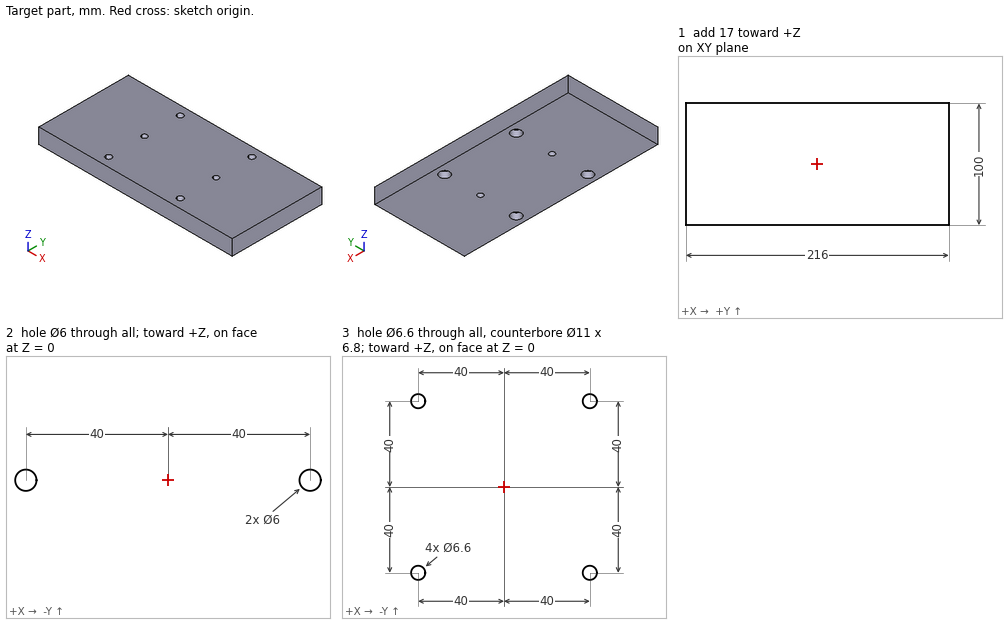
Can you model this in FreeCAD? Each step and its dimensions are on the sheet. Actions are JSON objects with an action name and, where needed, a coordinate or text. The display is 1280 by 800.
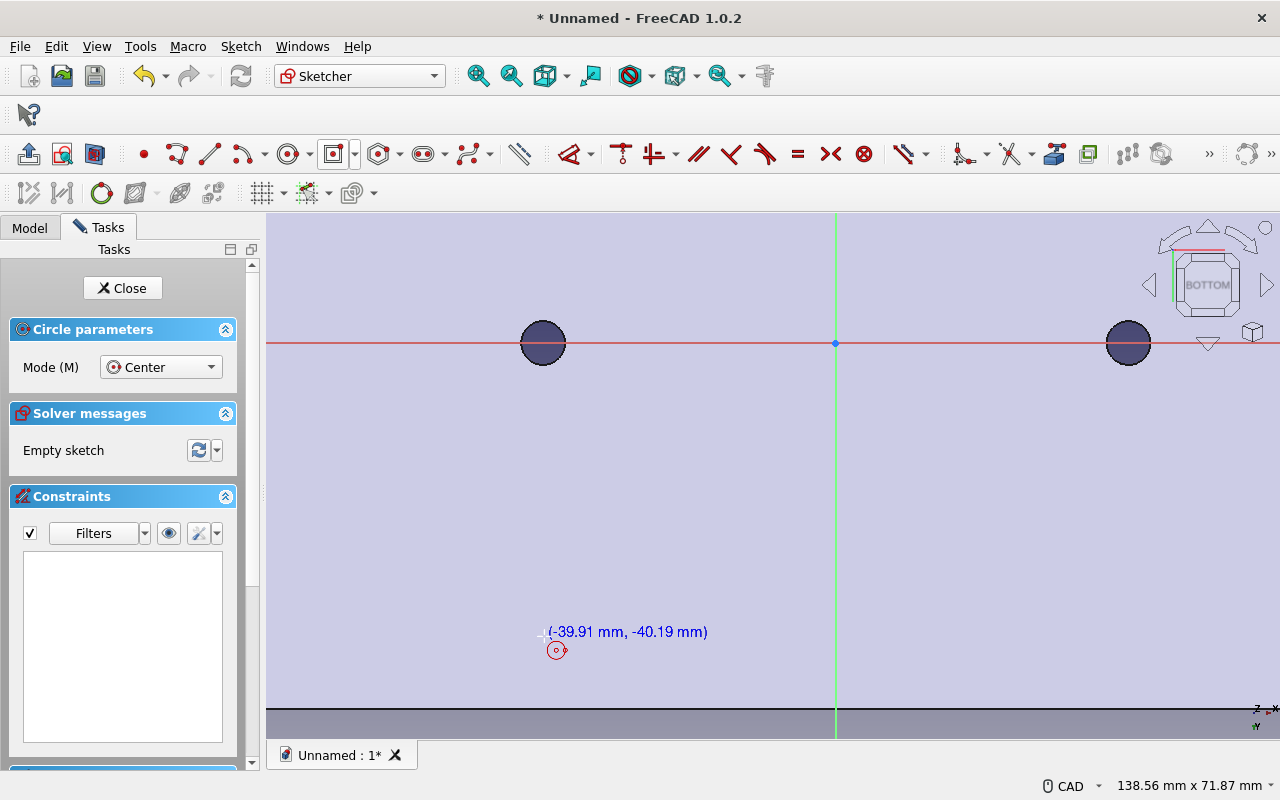
{"action": "left_click", "coordinate": [543, 636]}
{"action": "mouse_move", "coordinate": [560, 619]}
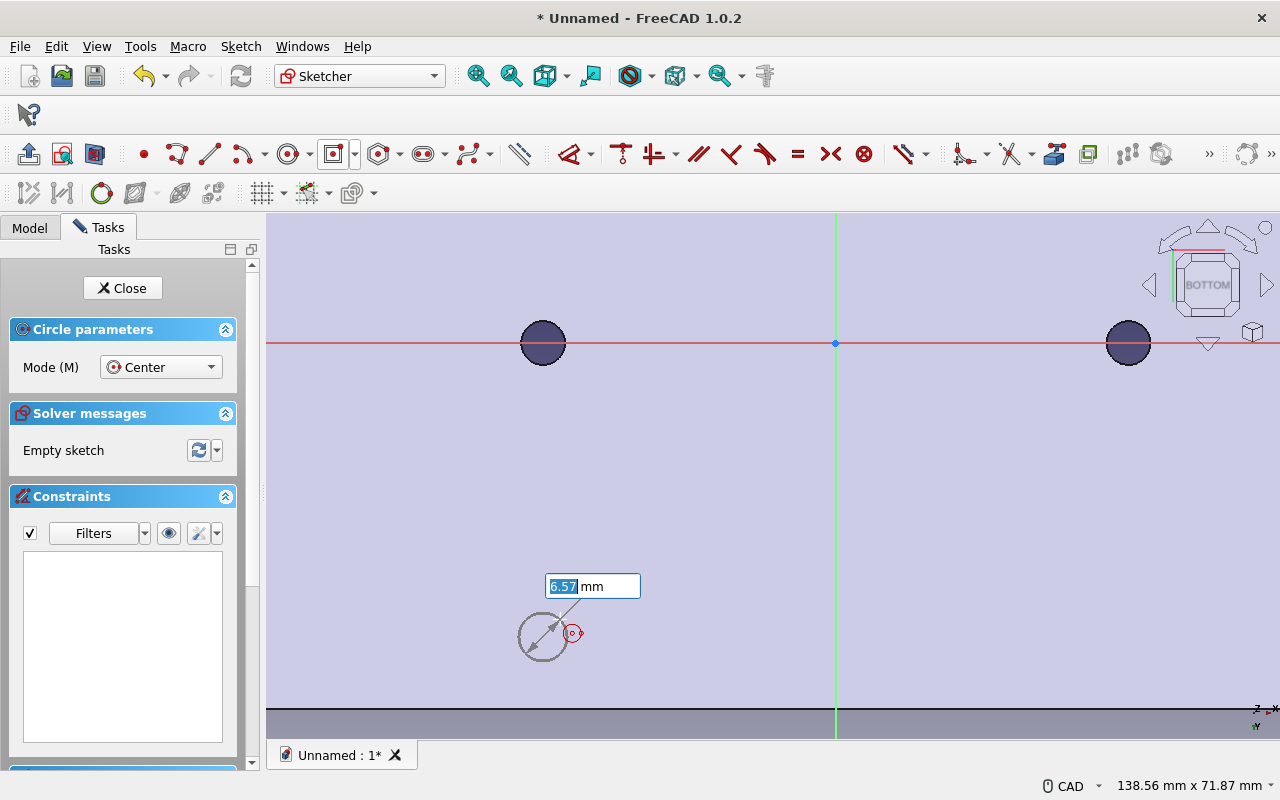
{"action": "type", "text": "6.6"}
{"action": "key", "text": "Return"}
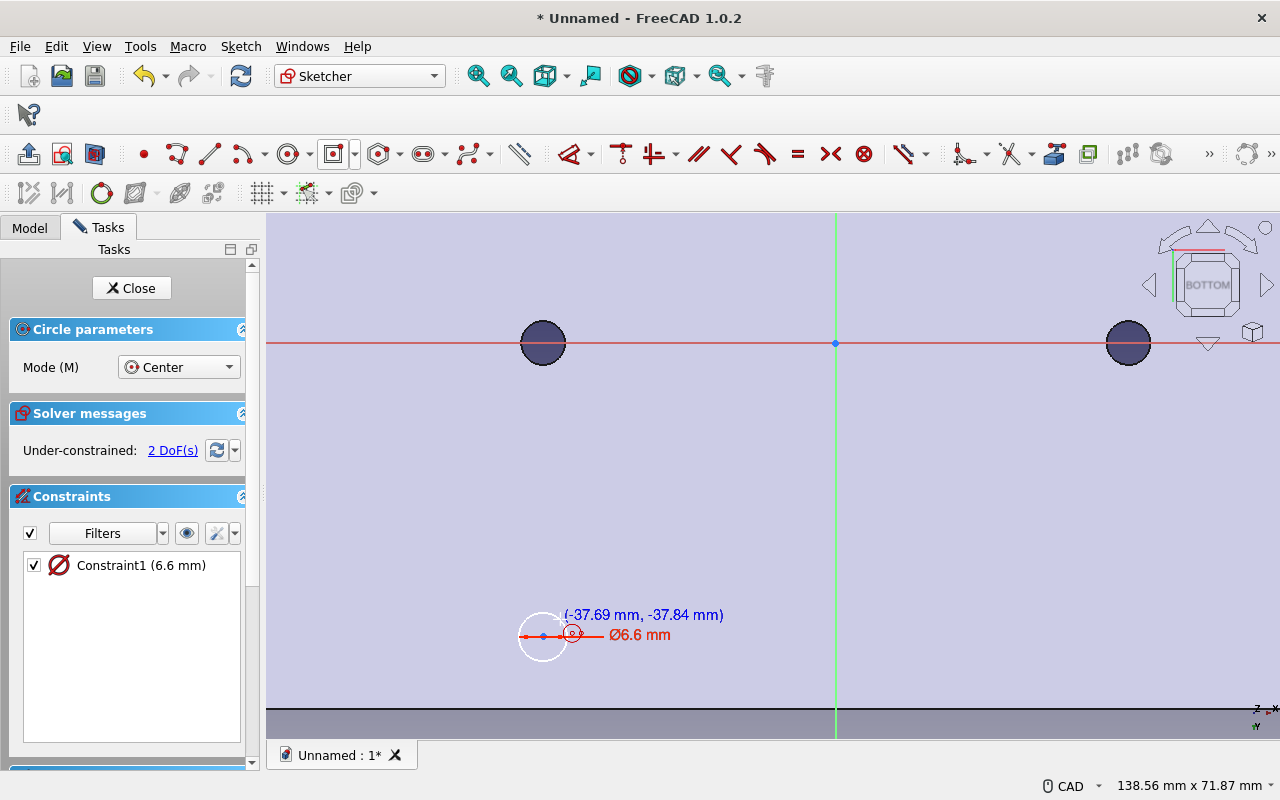
{"action": "scroll", "coordinate": [545, 638], "scroll_direction": "down", "scroll_amount": 3}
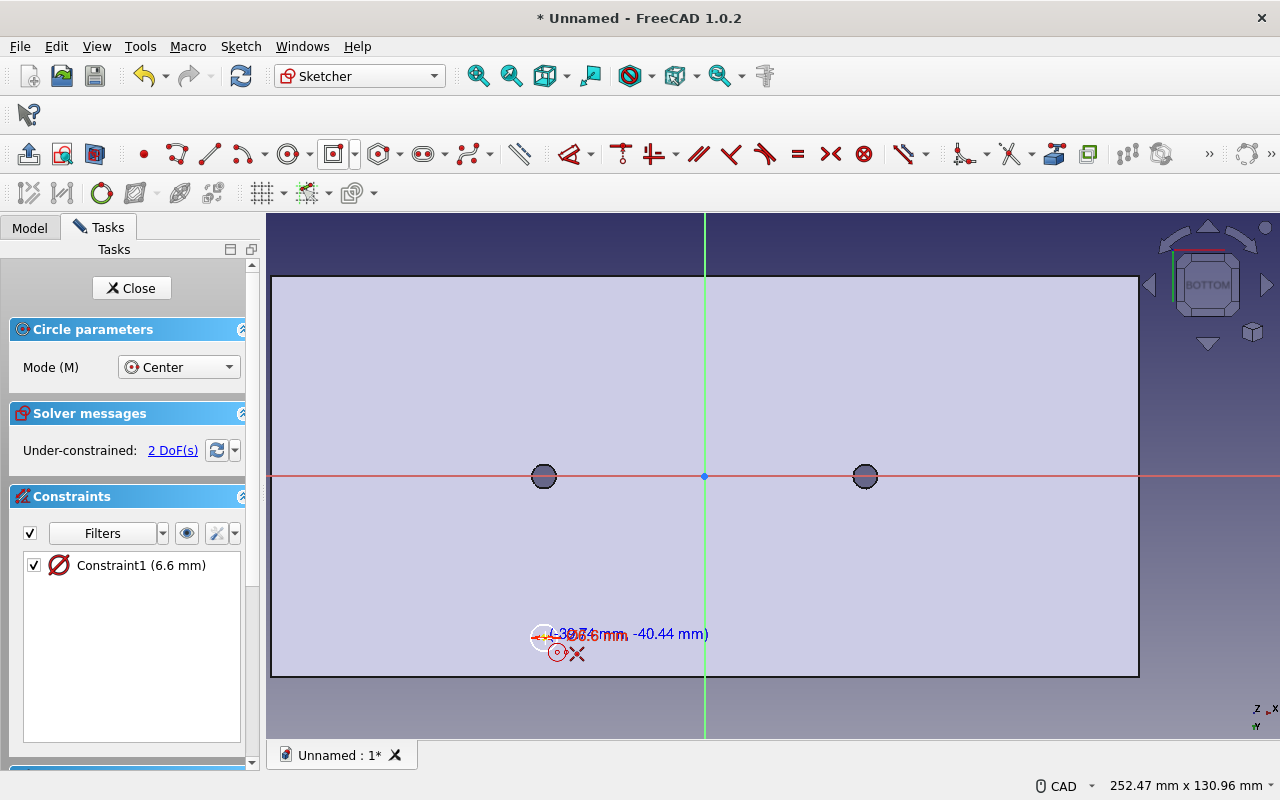
{"action": "scroll", "coordinate": [544, 316], "scroll_direction": "up", "scroll_amount": 3}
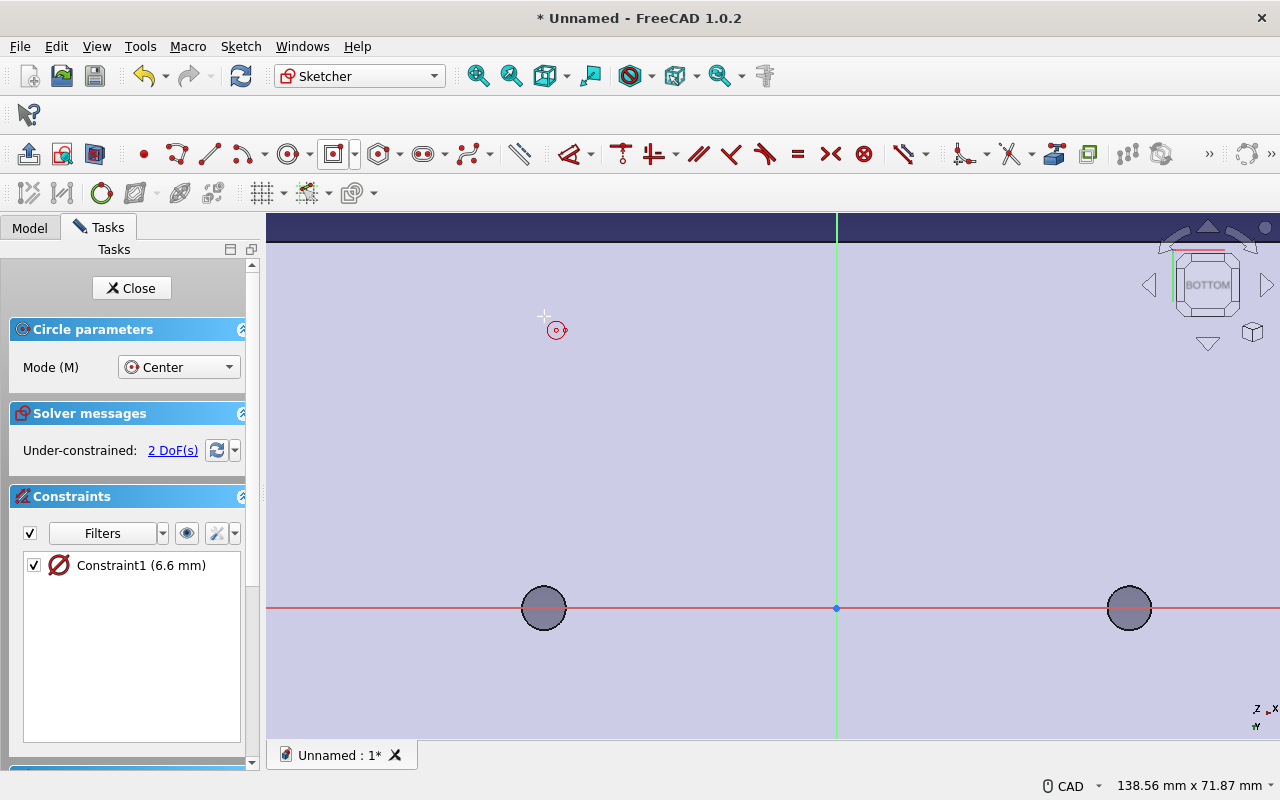
{"action": "left_click", "coordinate": [544, 316]}
{"action": "mouse_move", "coordinate": [561, 298]}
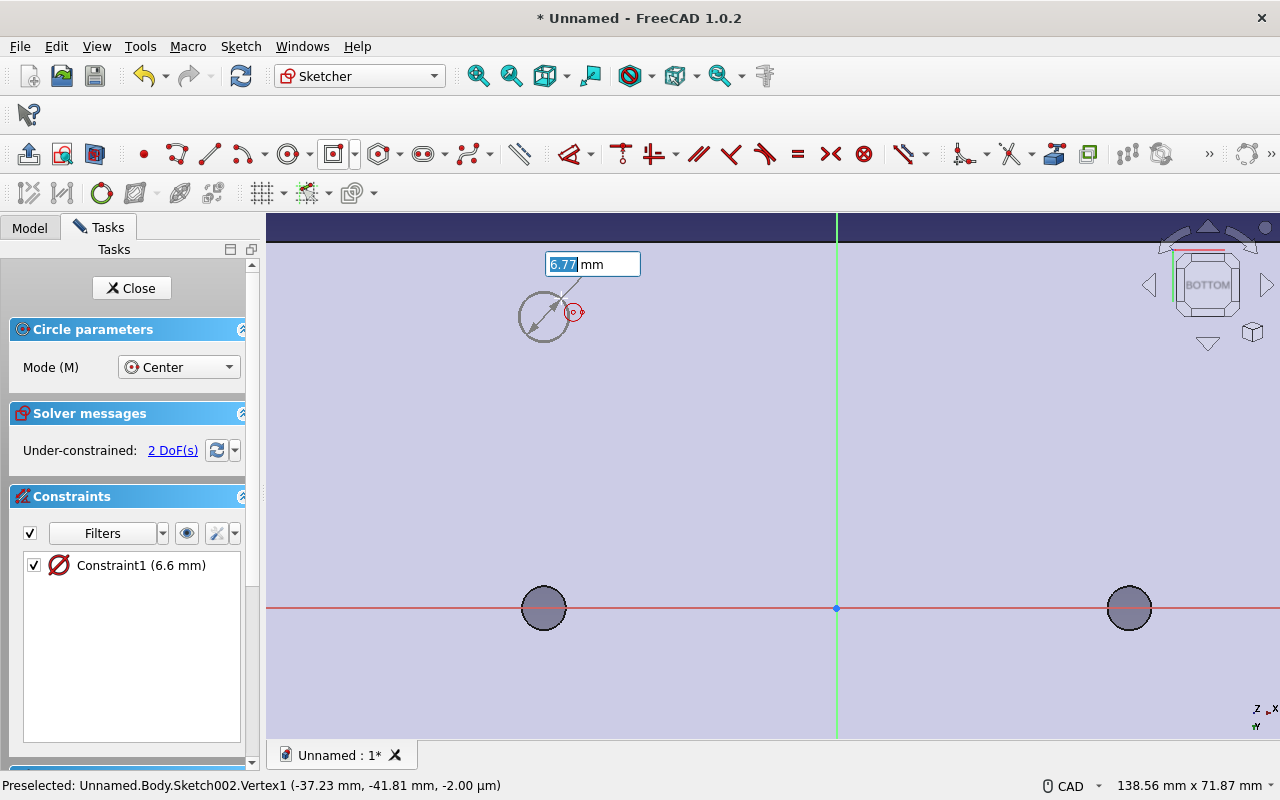
{"action": "type", "text": "6.6"}
{"action": "key", "text": "Return"}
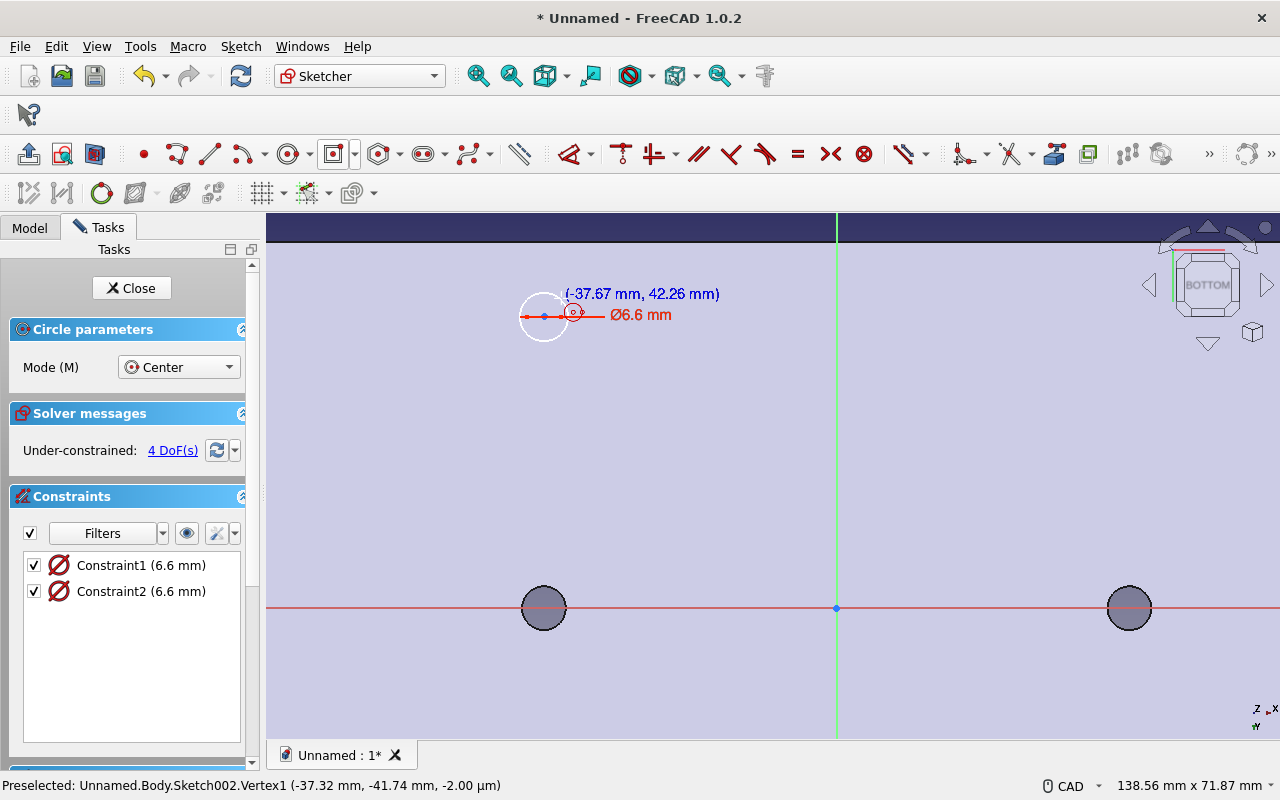
{"action": "scroll", "coordinate": [544, 315], "scroll_direction": "down", "scroll_amount": 3}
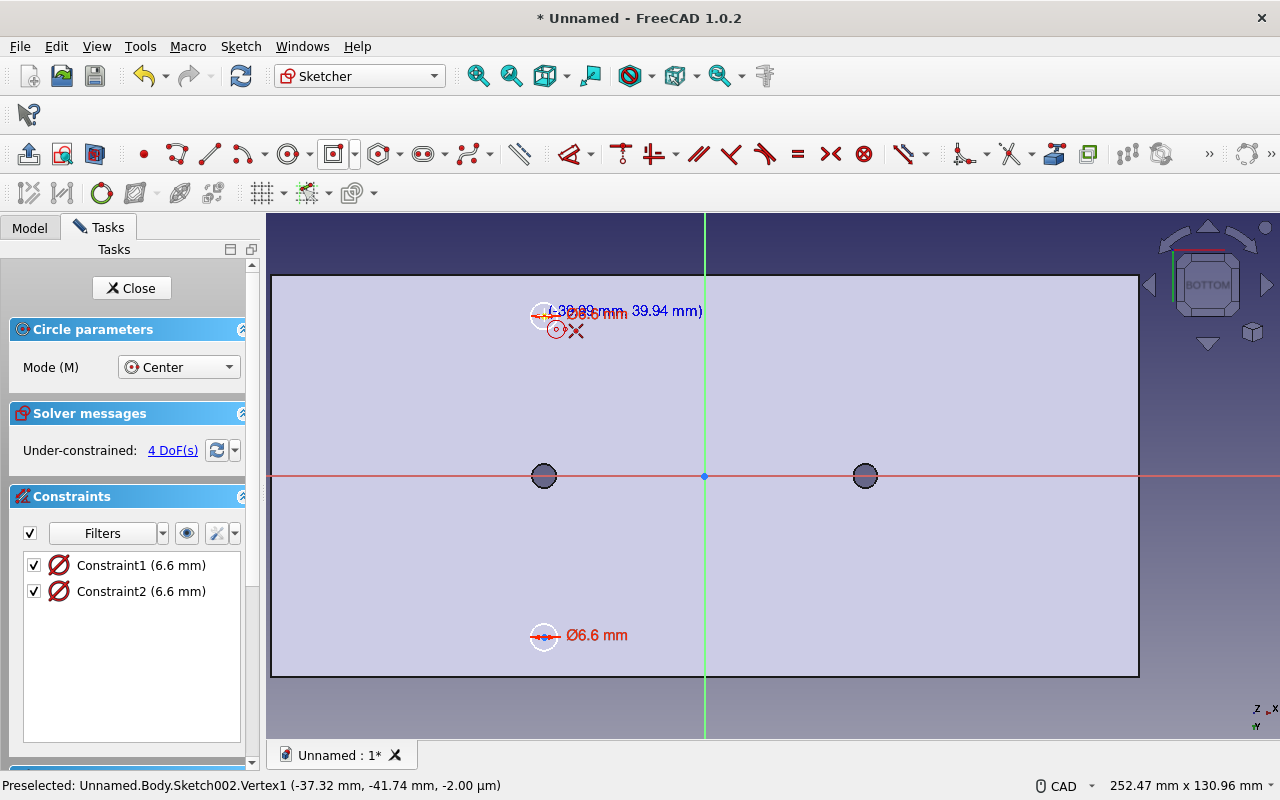
{"action": "scroll", "coordinate": [865, 315], "scroll_direction": "up", "scroll_amount": 3}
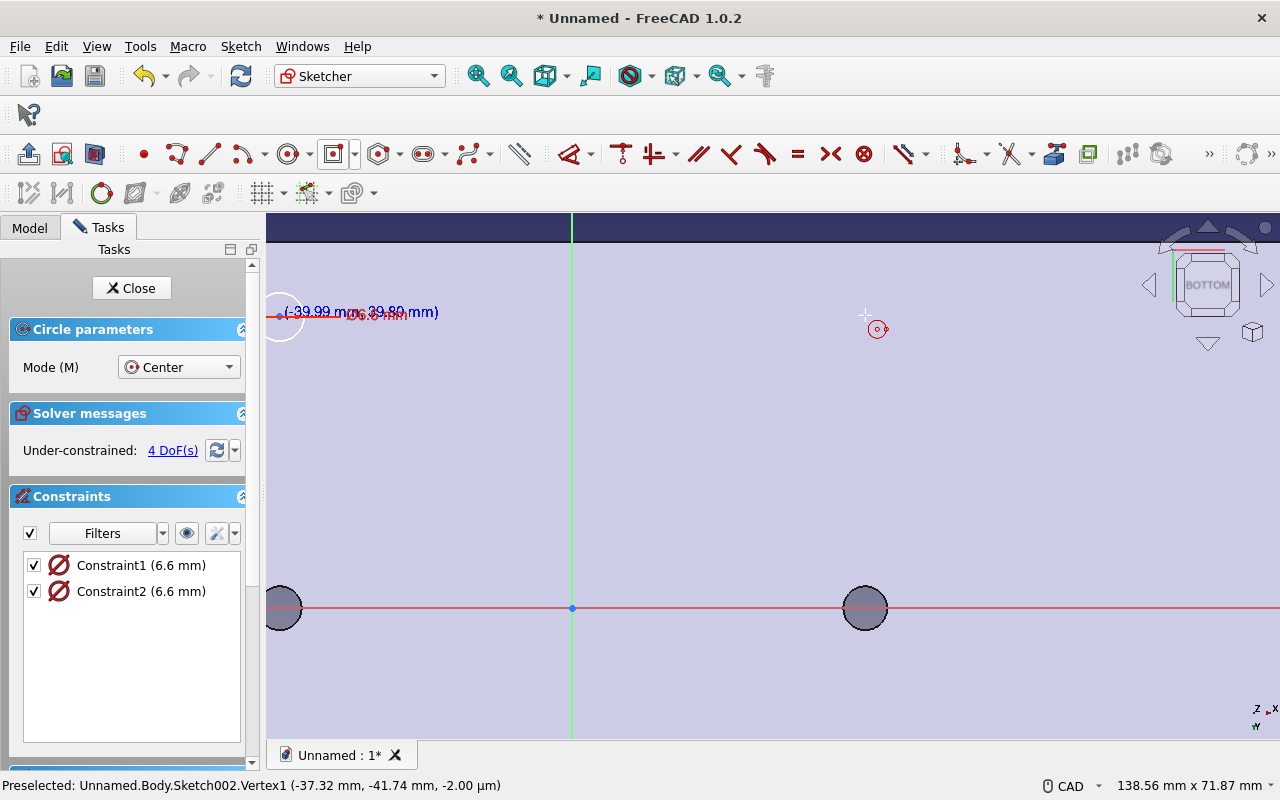
{"action": "left_click", "coordinate": [865, 316]}
{"action": "mouse_move", "coordinate": [882, 298]}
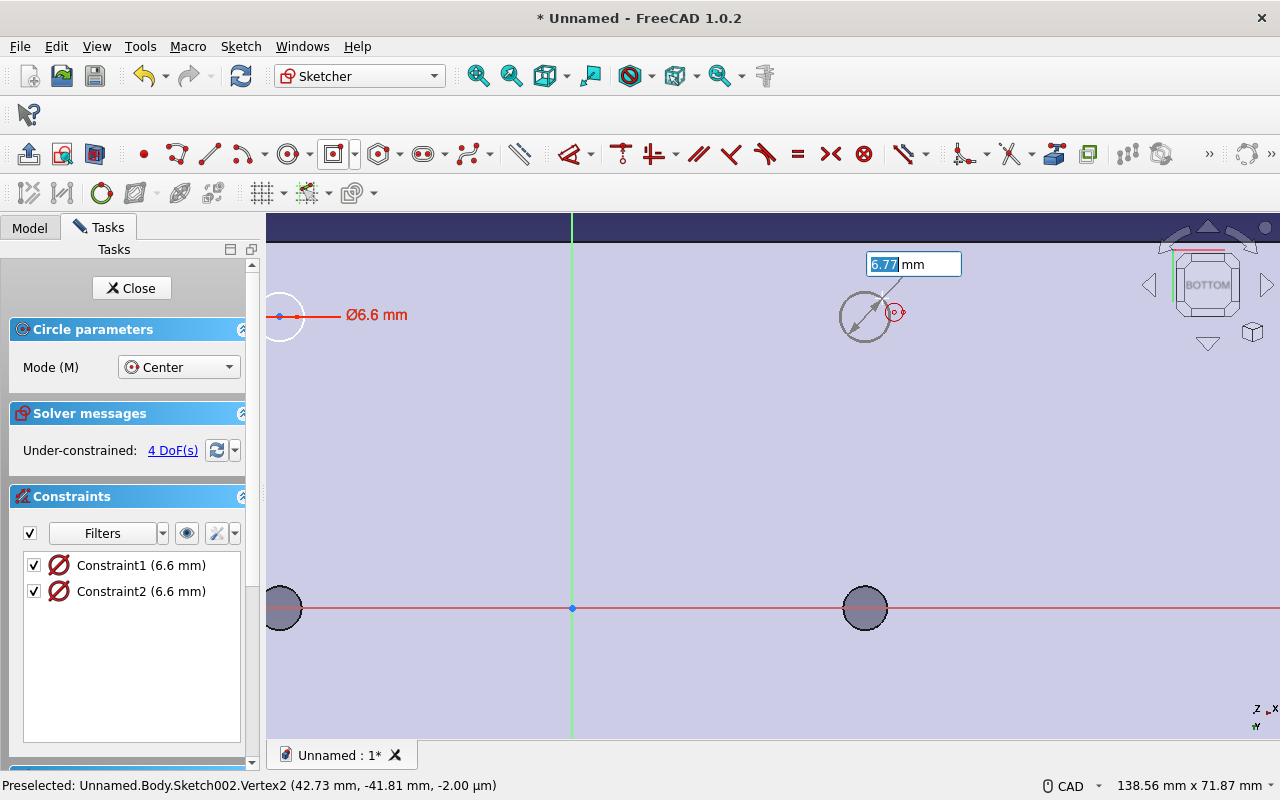
{"action": "type", "text": "6.6"}
{"action": "key", "text": "Return"}